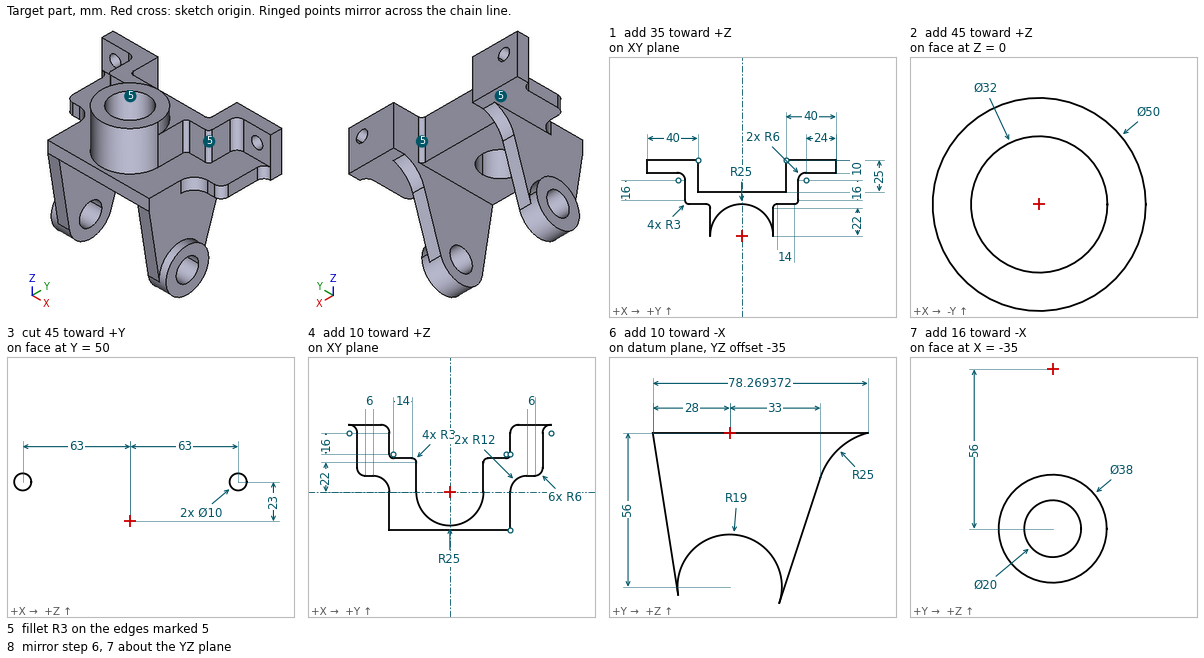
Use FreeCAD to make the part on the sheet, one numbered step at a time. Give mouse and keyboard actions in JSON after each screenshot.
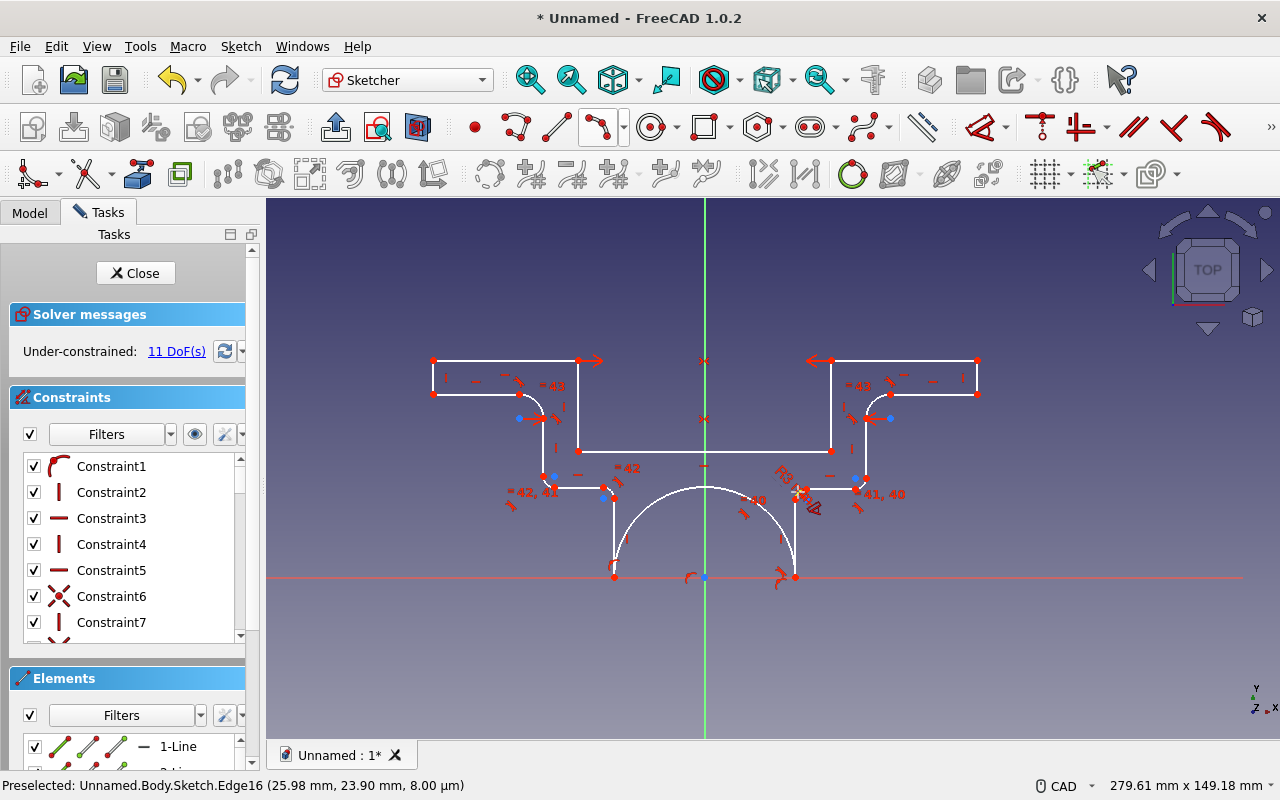
{"action": "scroll", "coordinate": [879, 397], "scroll_direction": "up", "scroll_amount": 4}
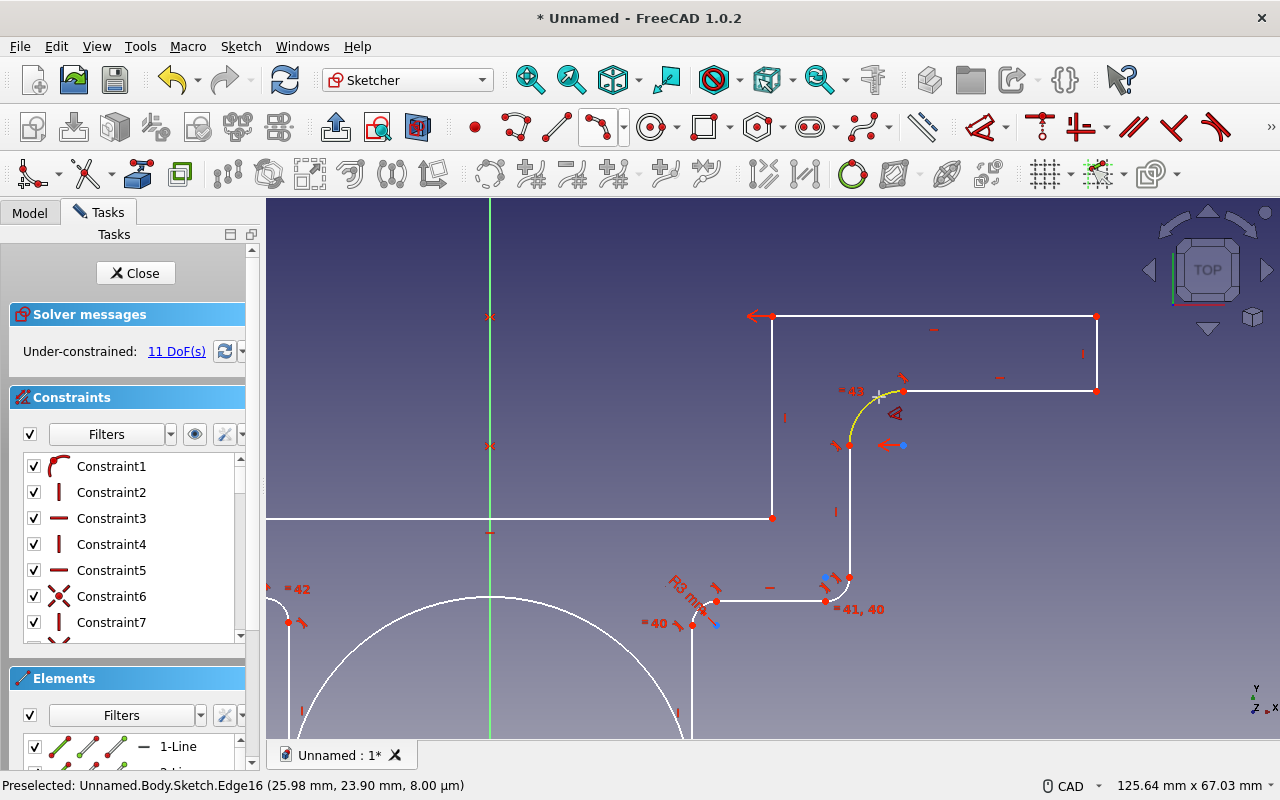
{"action": "left_click", "coordinate": [879, 397]}
{"action": "left_click", "coordinate": [864, 369]}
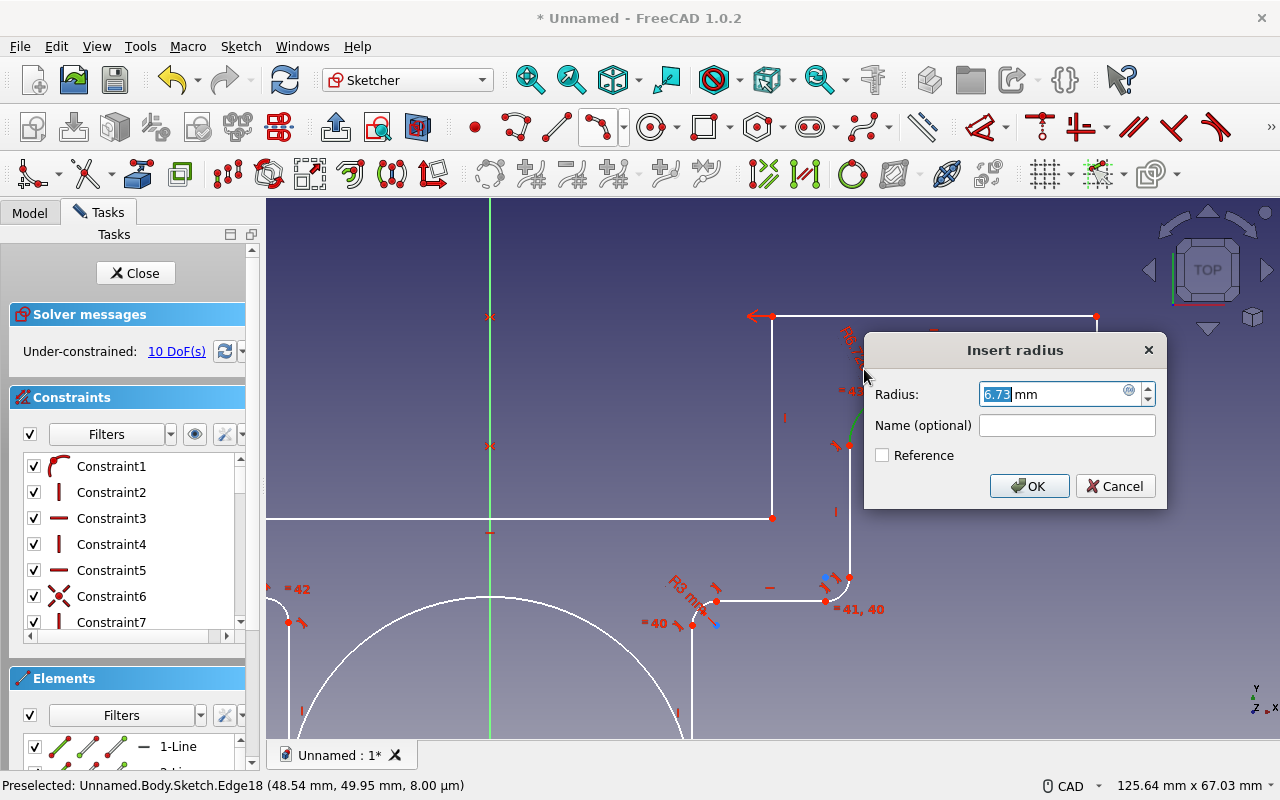
{"action": "type", "text": "6"}
{"action": "key", "text": "Return"}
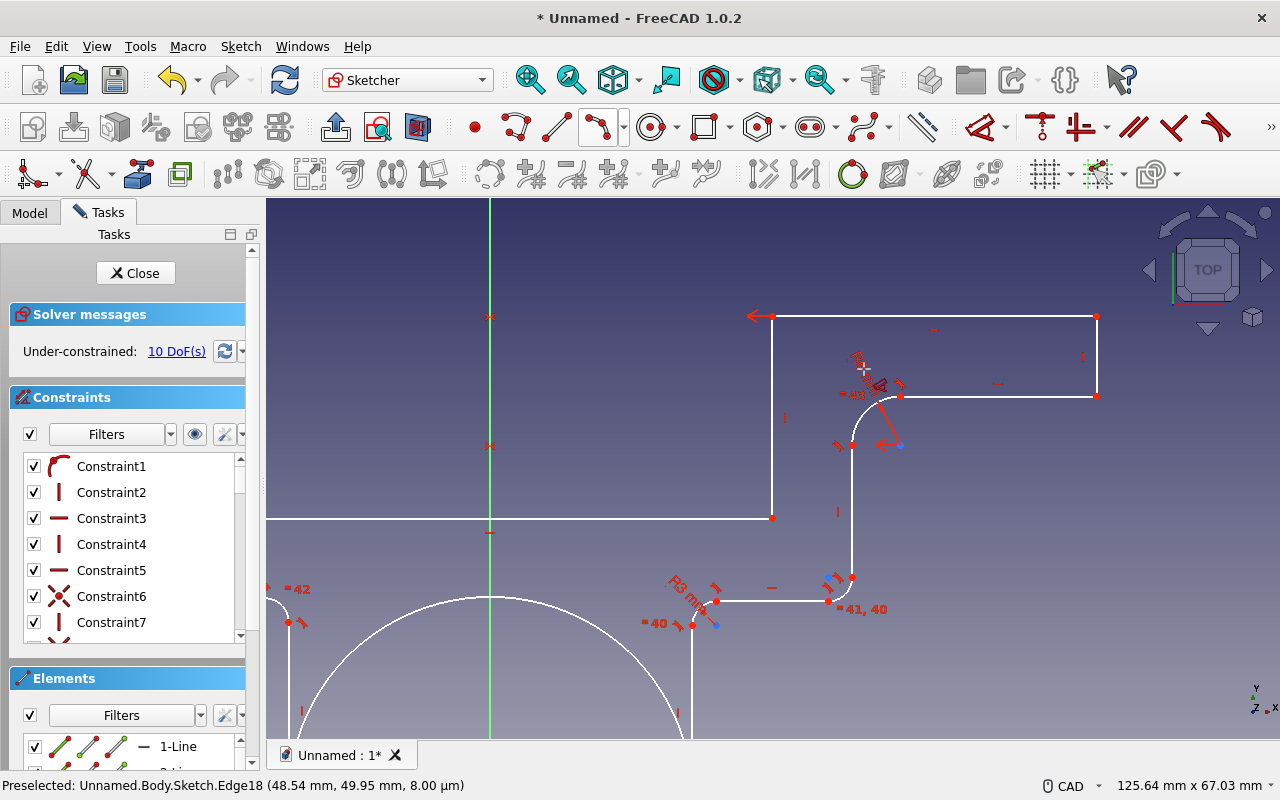
{"action": "left_click", "coordinate": [609, 635]}
{"action": "left_click", "coordinate": [520, 566]}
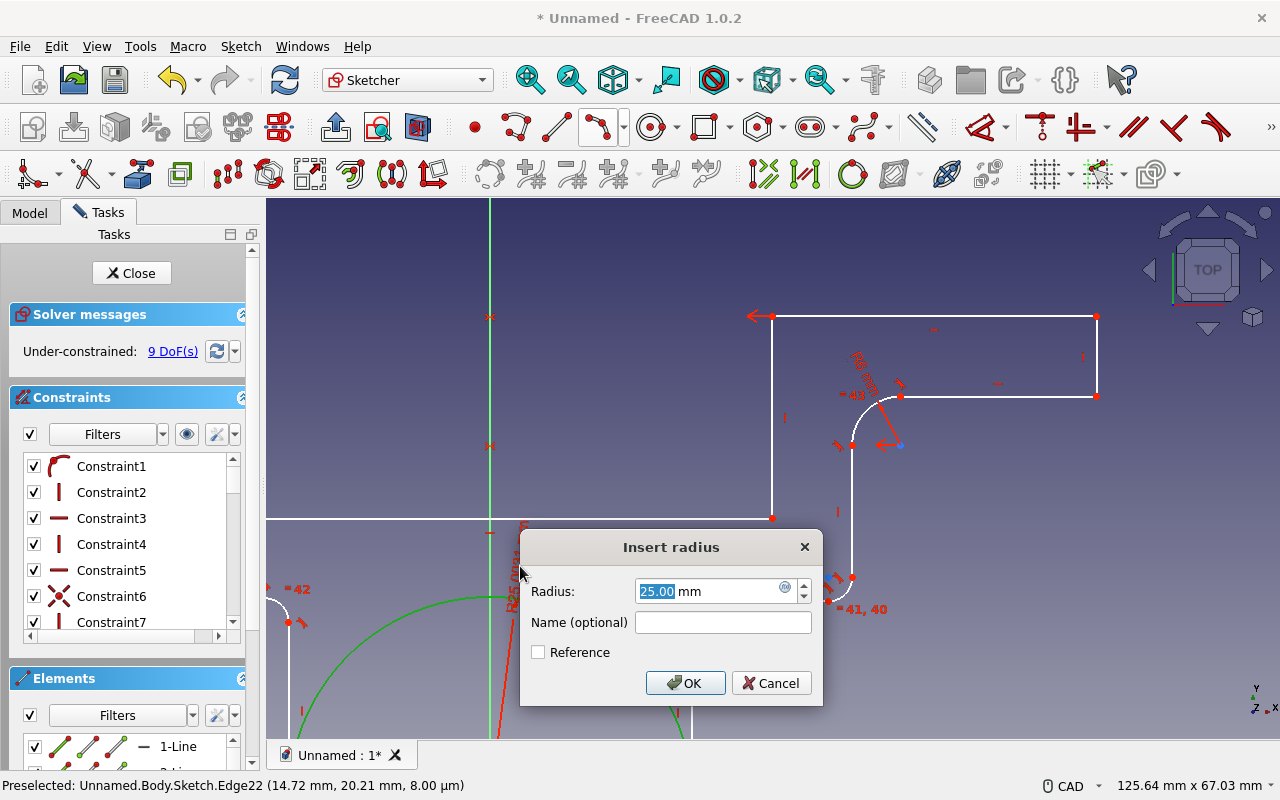
{"action": "type", "text": "25"}
{"action": "key", "text": "Return"}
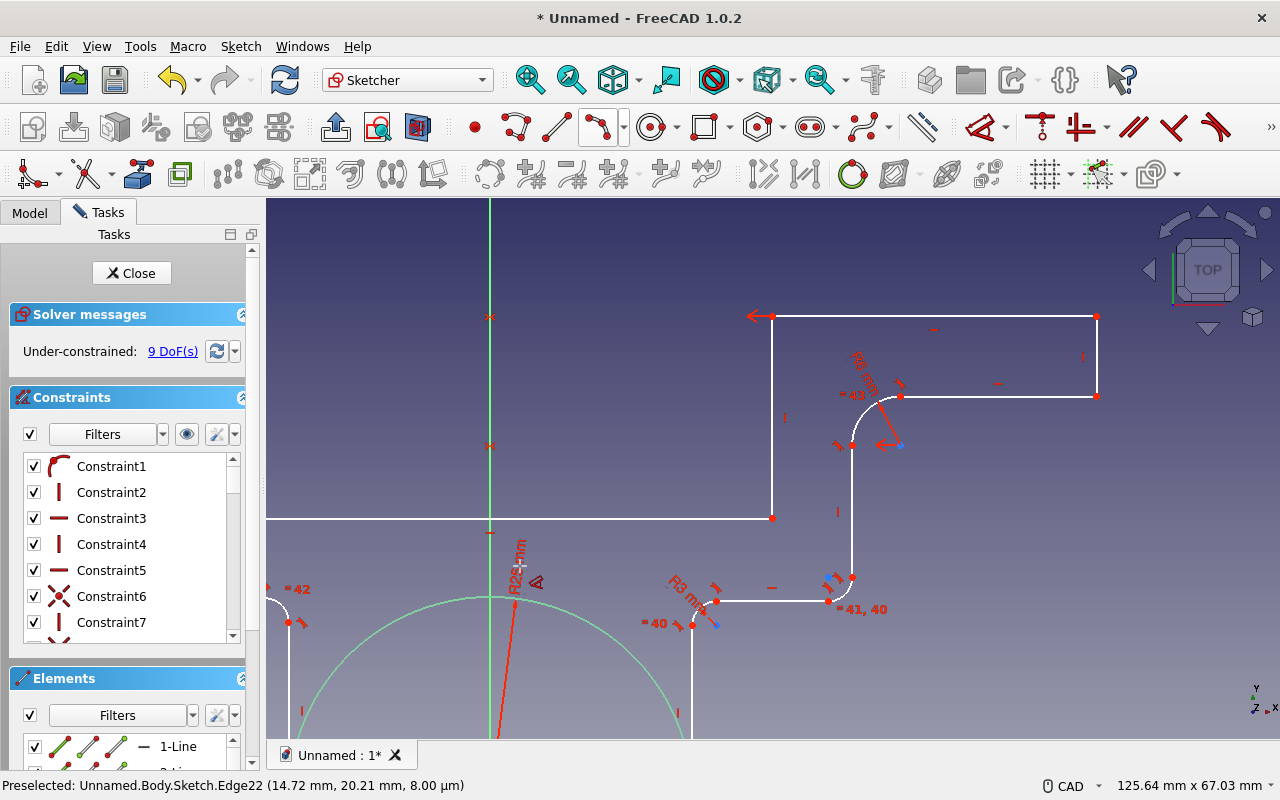
{"action": "left_click", "coordinate": [692, 678]}
{"action": "left_click", "coordinate": [726, 668]}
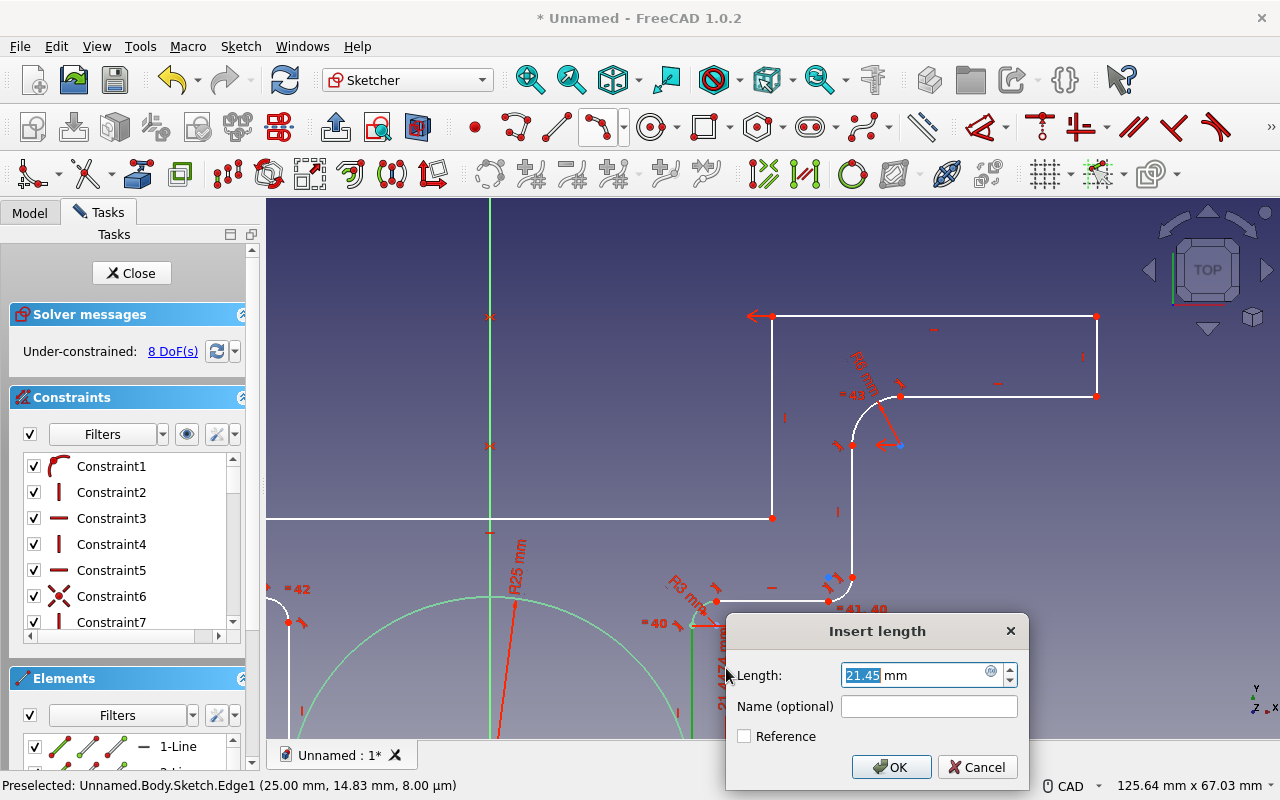
{"action": "type", "text": "22"}
{"action": "key", "text": "Return"}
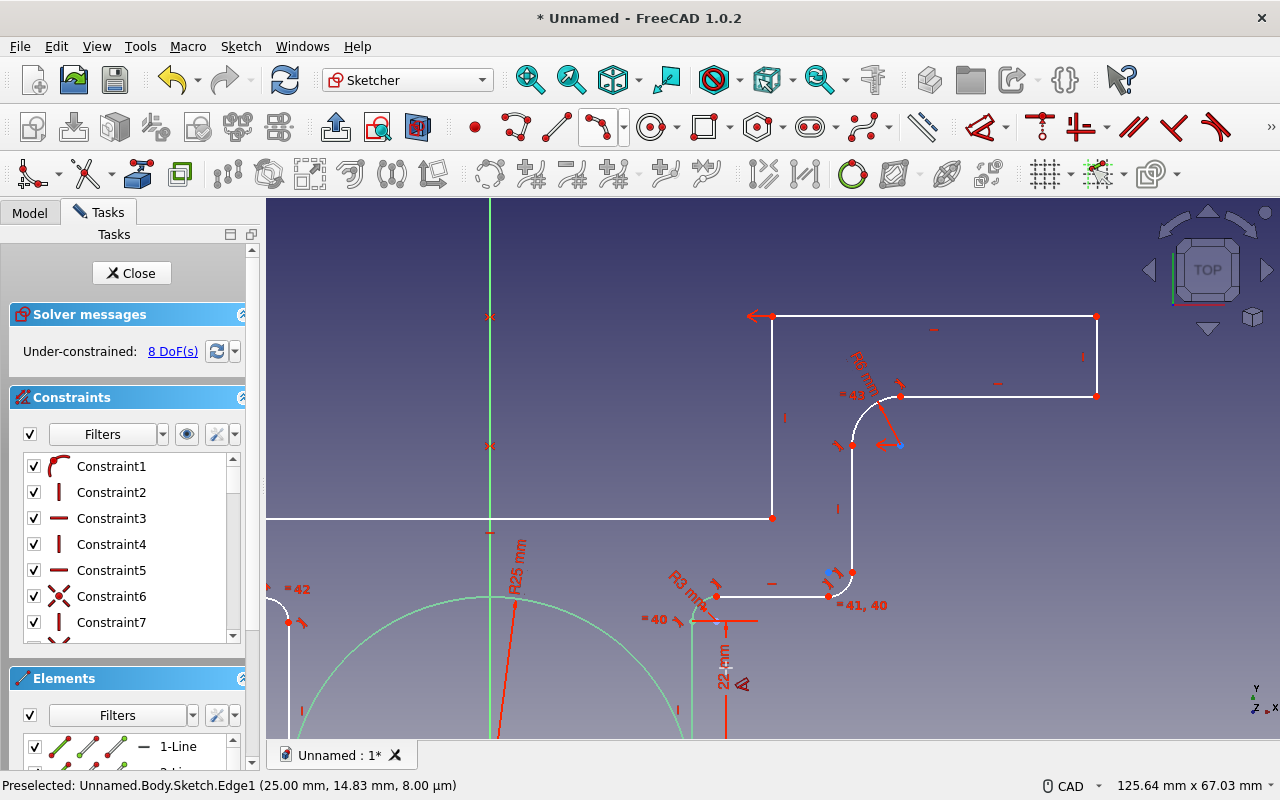
{"action": "left_click", "coordinate": [750, 597]}
{"action": "left_click", "coordinate": [772, 631]}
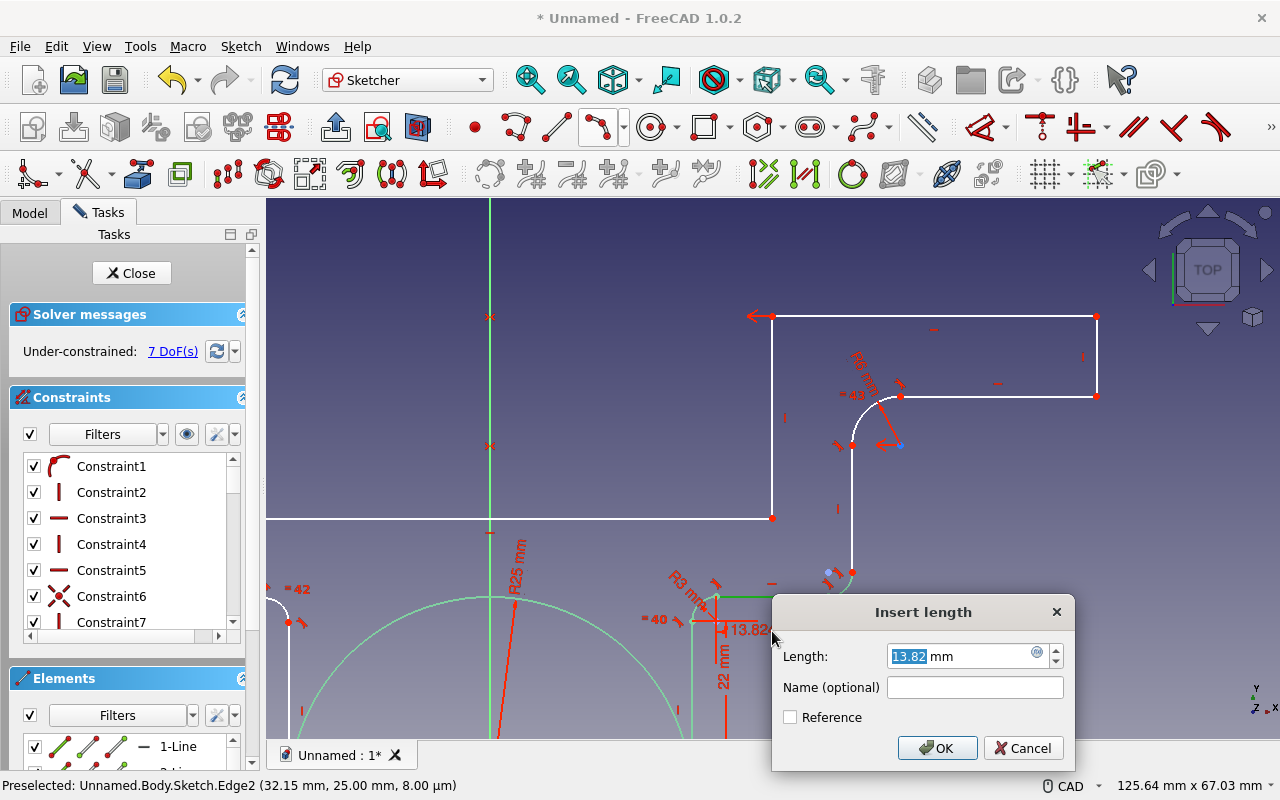
{"action": "type", "text": "14"}
{"action": "key", "text": "Return"}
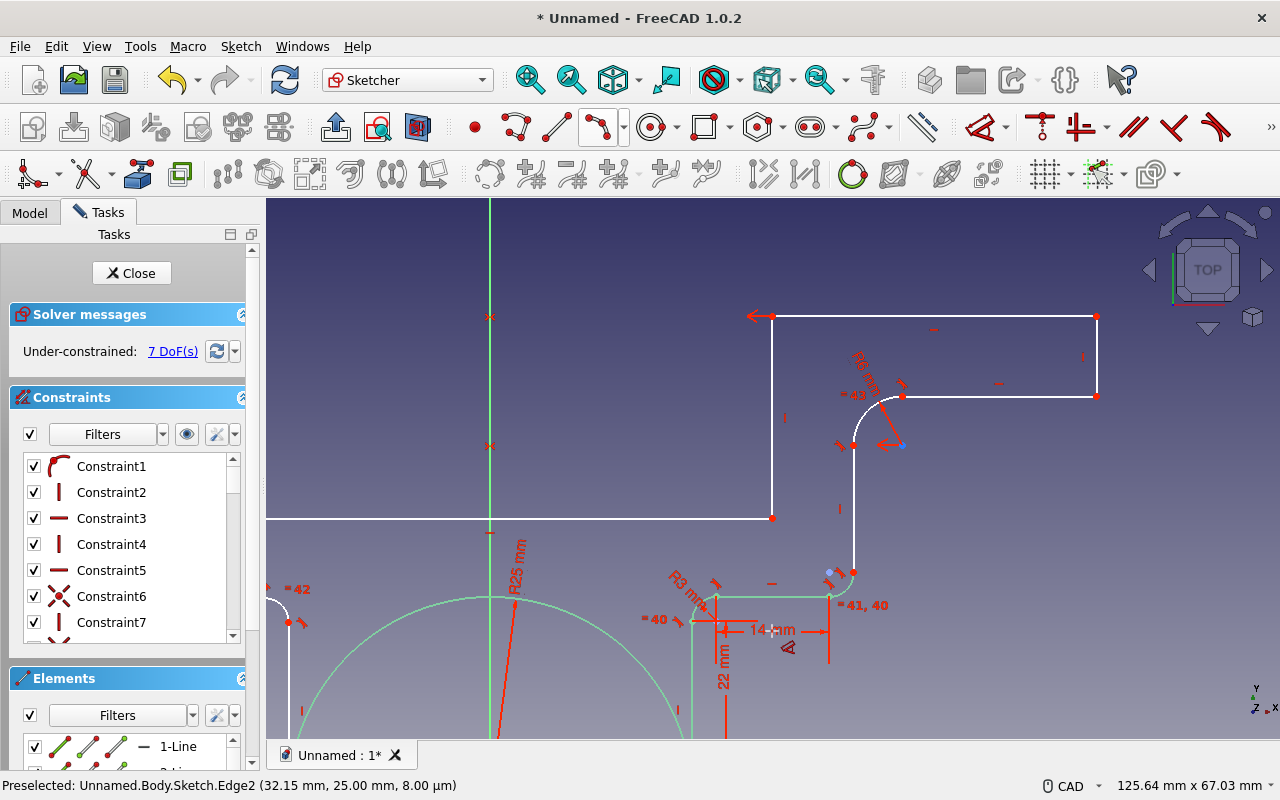
{"action": "left_click", "coordinate": [854, 534]}
{"action": "left_click", "coordinate": [888, 509]}